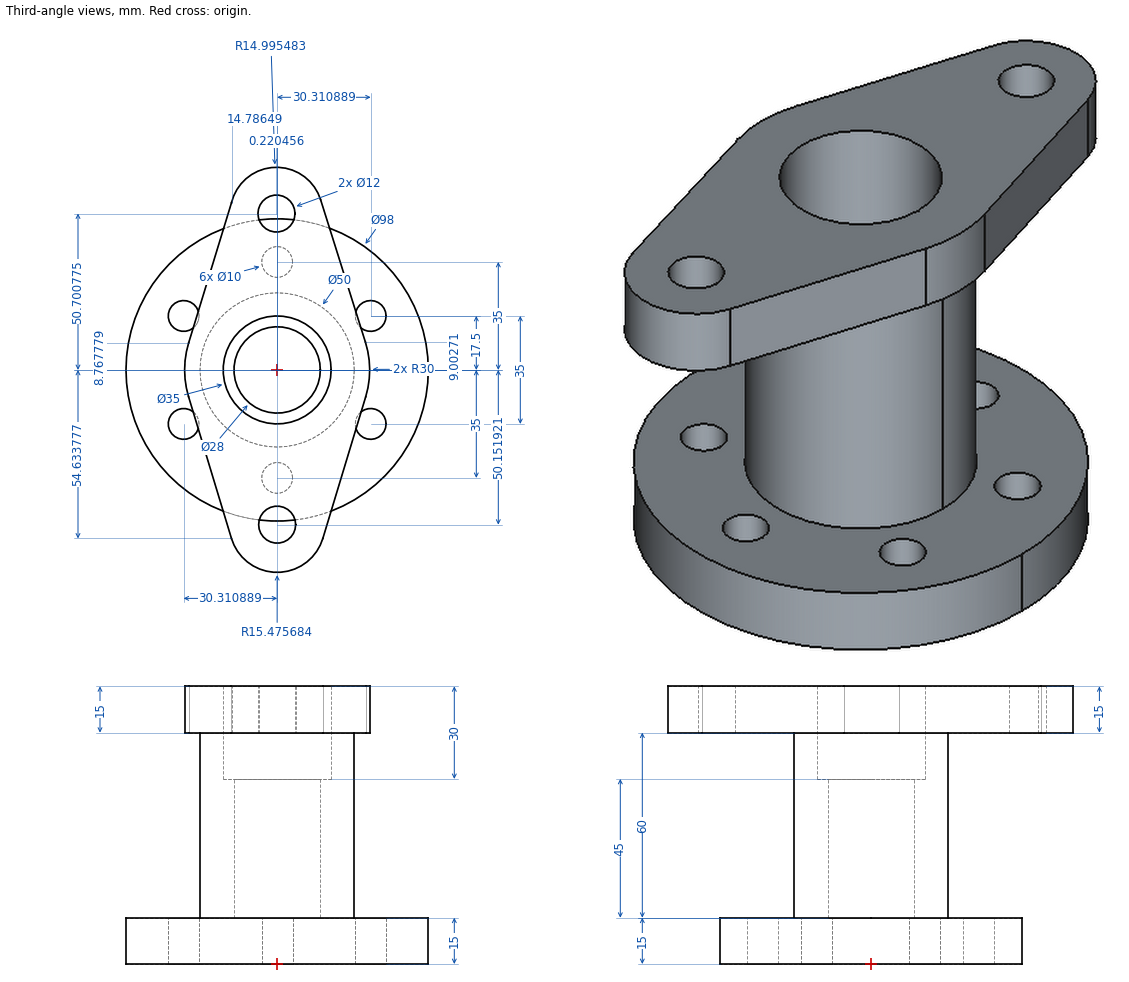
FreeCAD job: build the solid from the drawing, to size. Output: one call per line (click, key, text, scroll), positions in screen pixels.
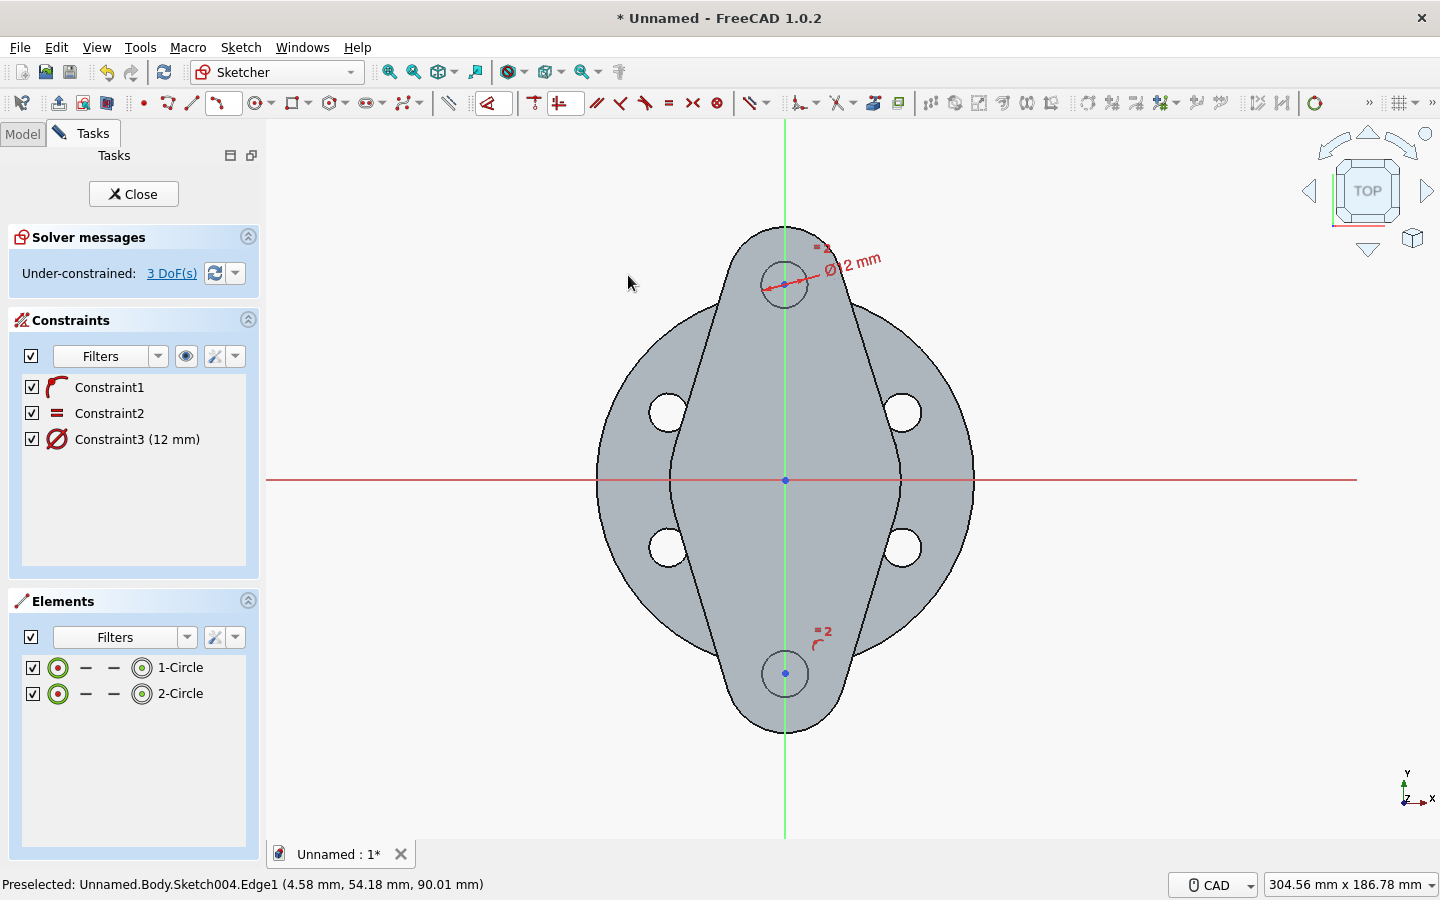
scroll(784, 285, up, 20)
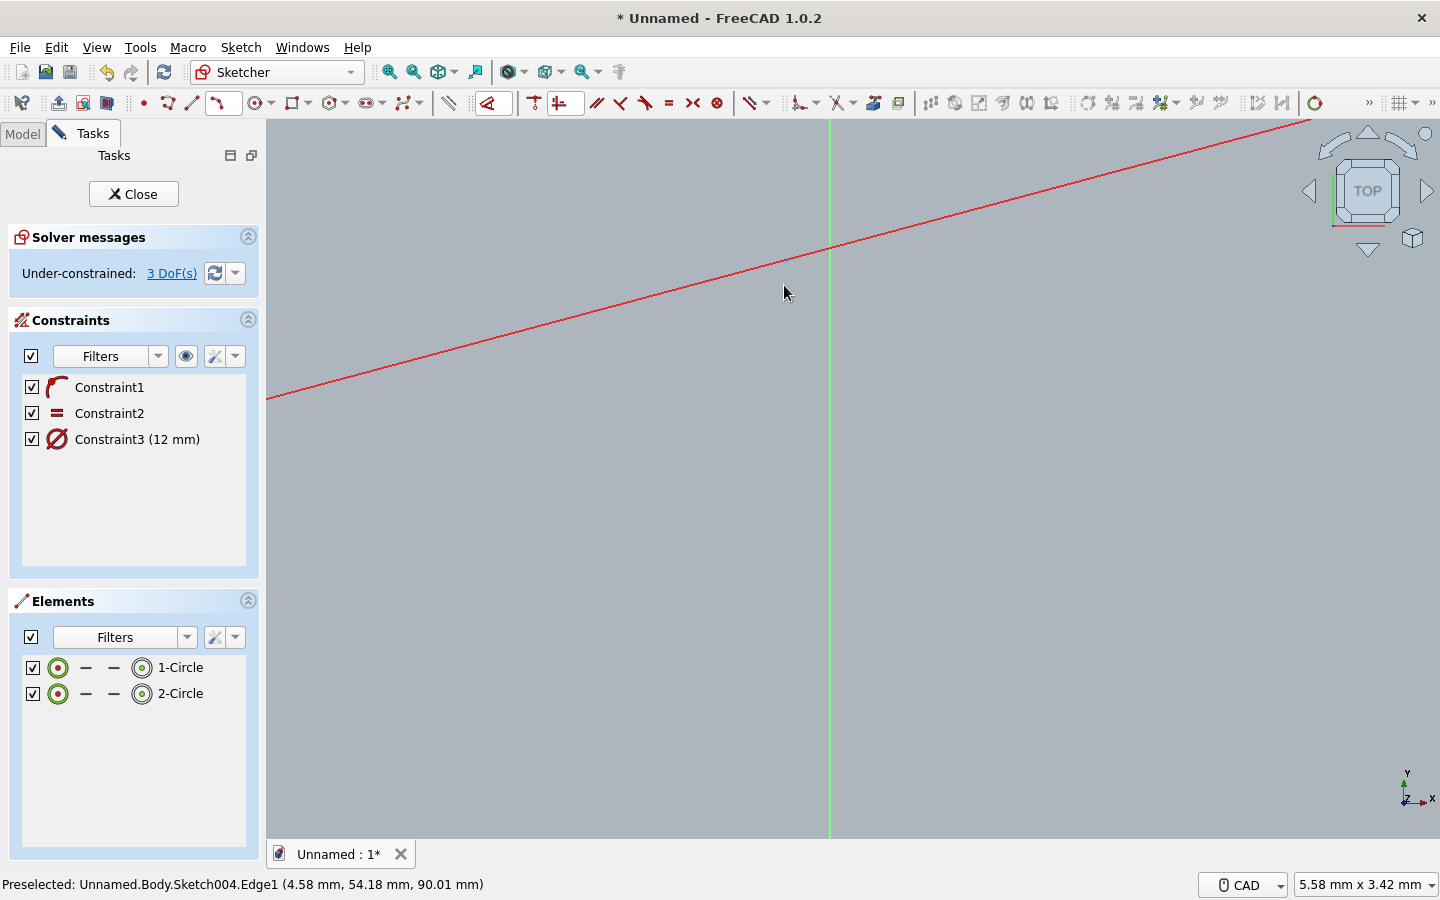
click(785, 260)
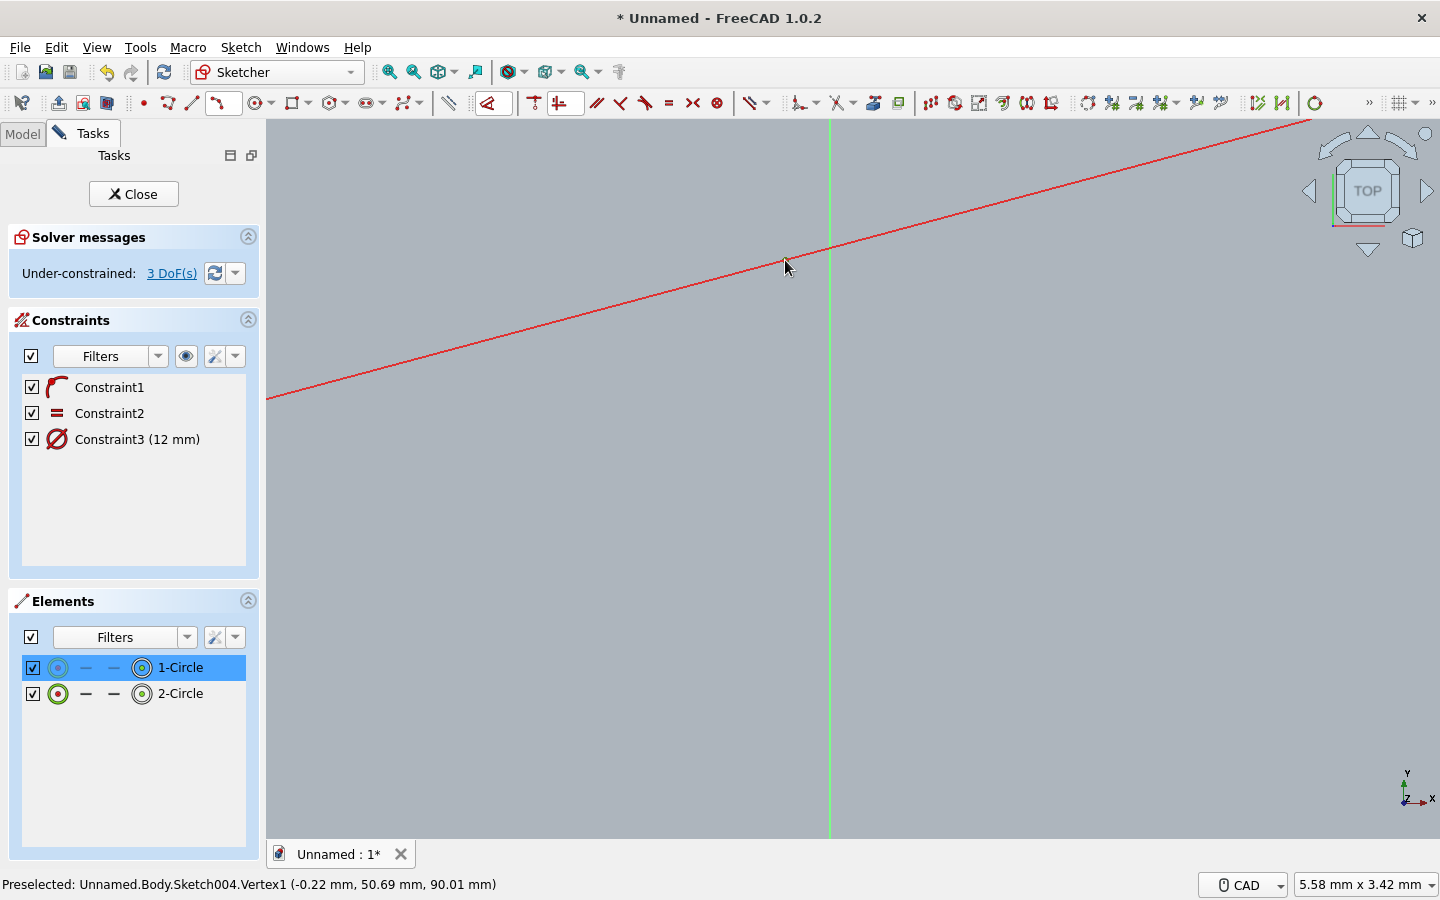
key(l)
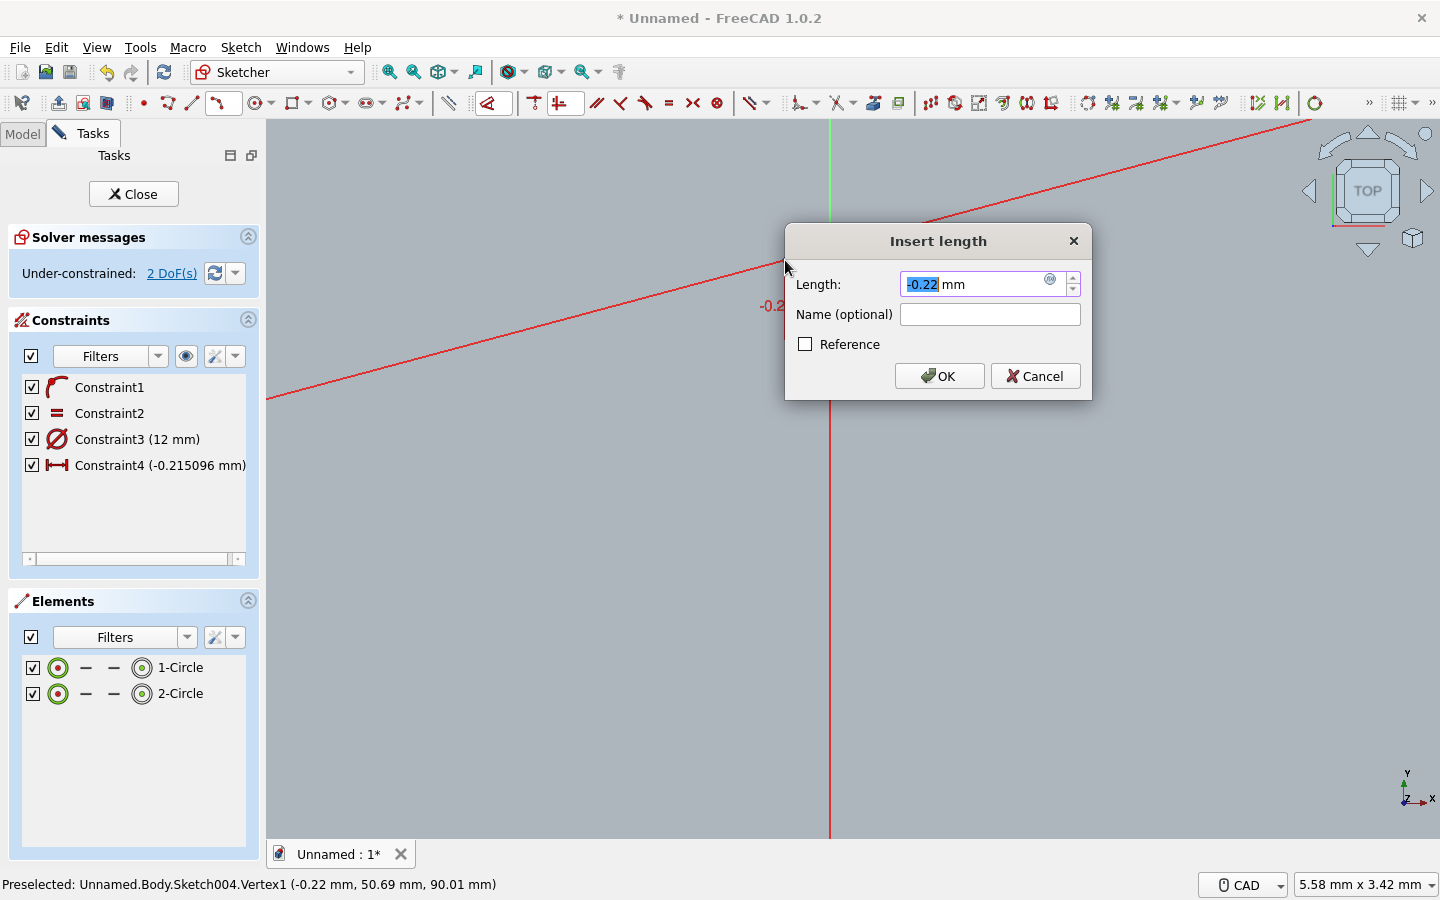
text(-0.220456)
key(Return)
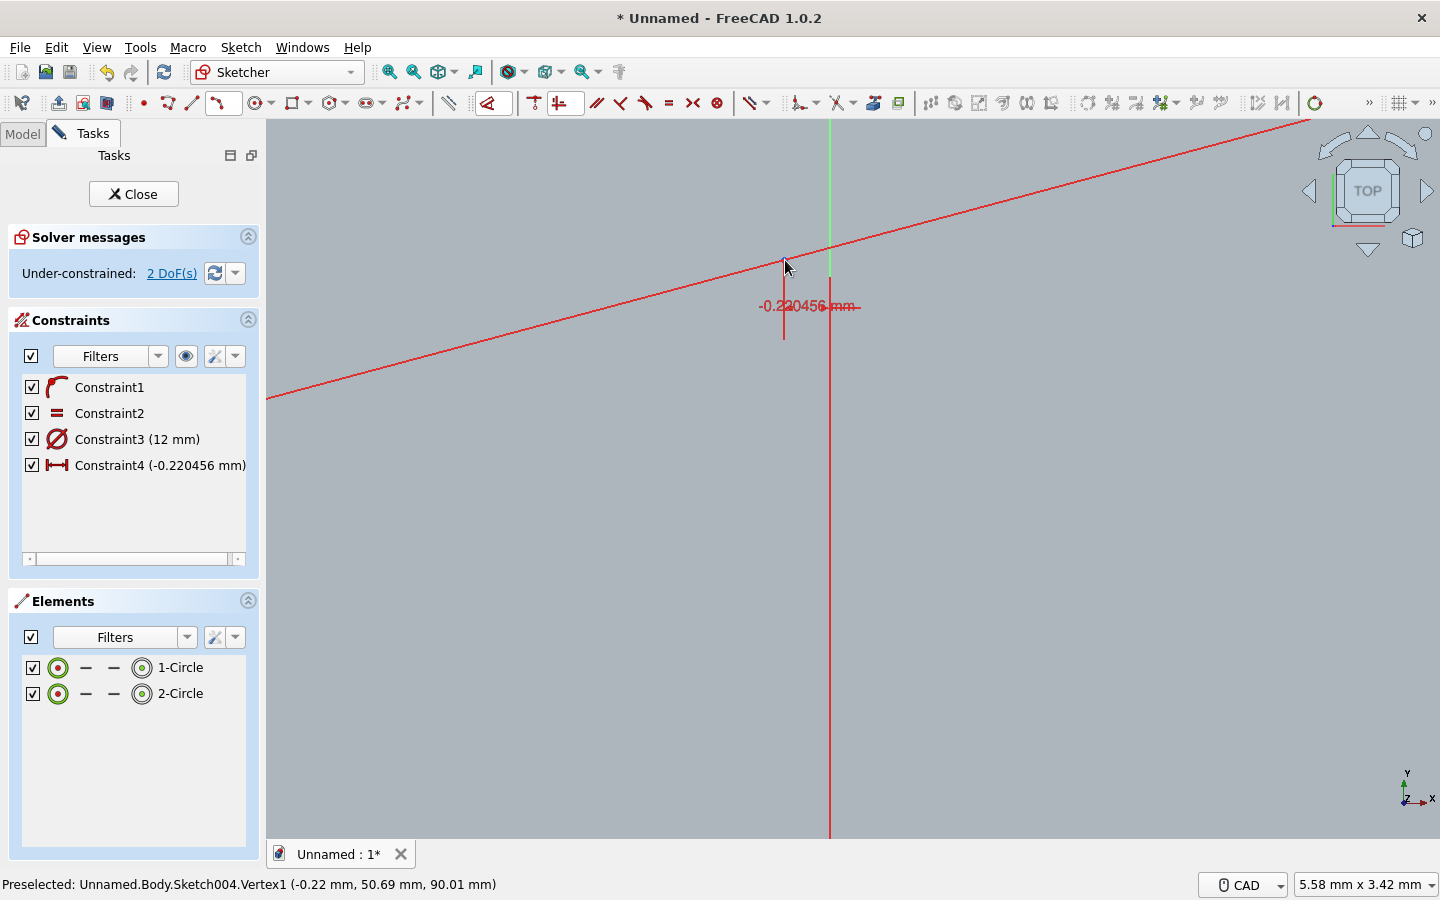
scroll(784, 479, down, 15)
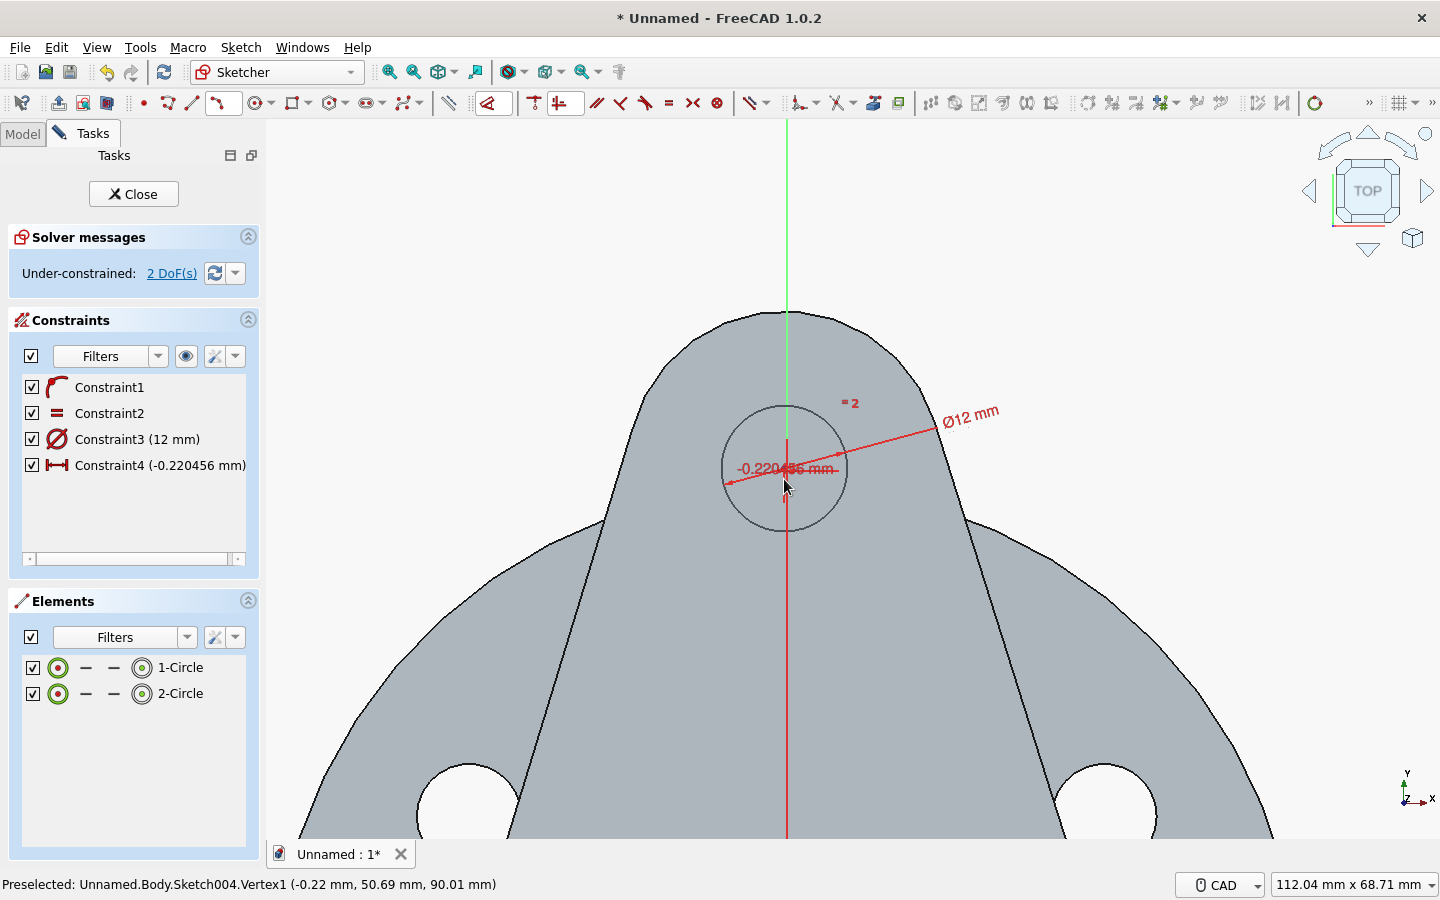
scroll(784, 178, down, 5)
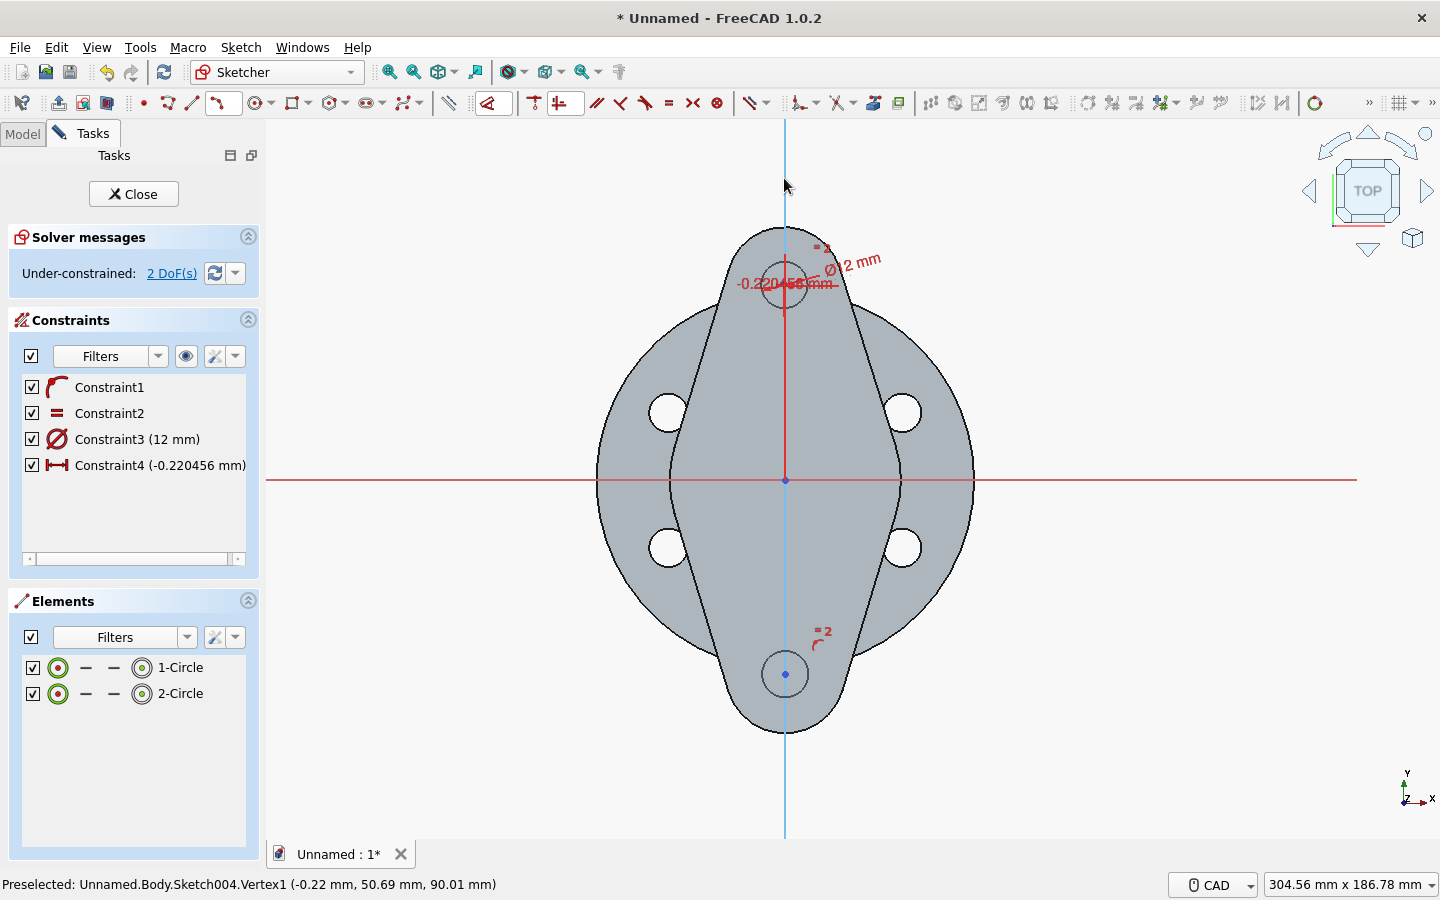
click(784, 285)